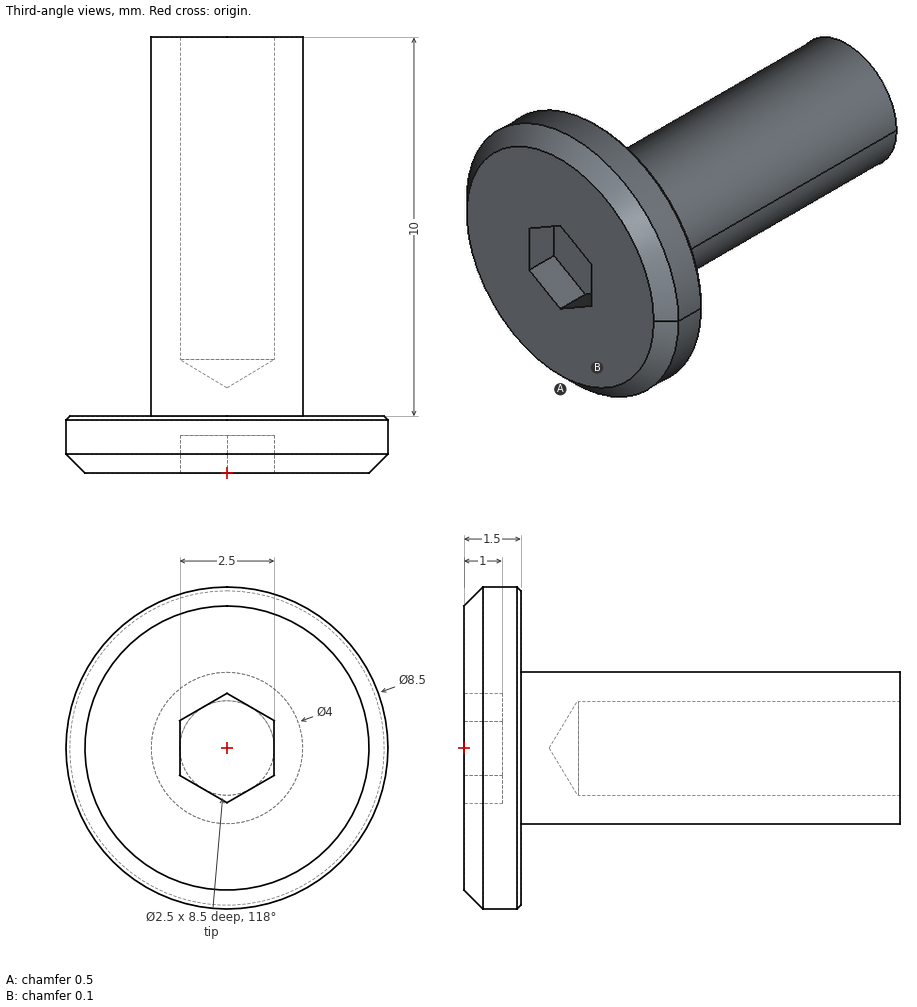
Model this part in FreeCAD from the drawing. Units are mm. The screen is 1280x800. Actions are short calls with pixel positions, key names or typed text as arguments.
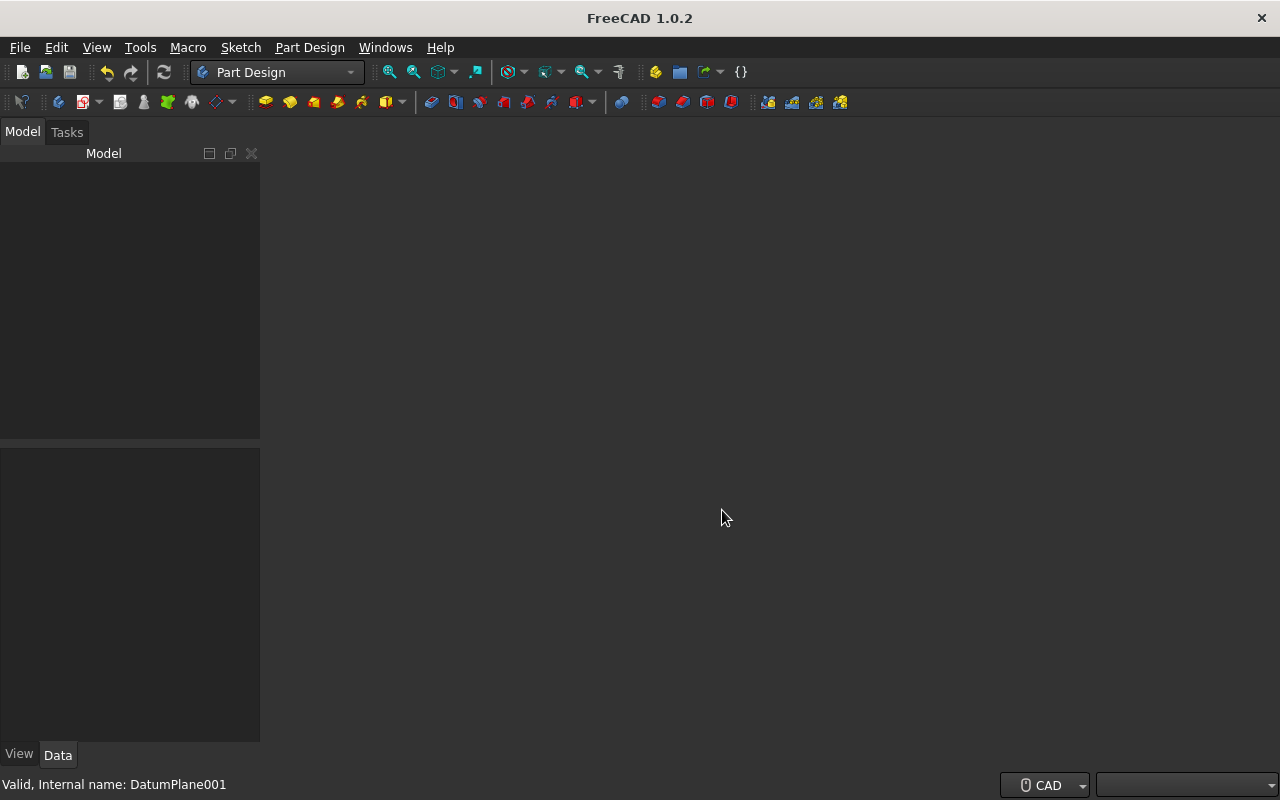
click(22, 72)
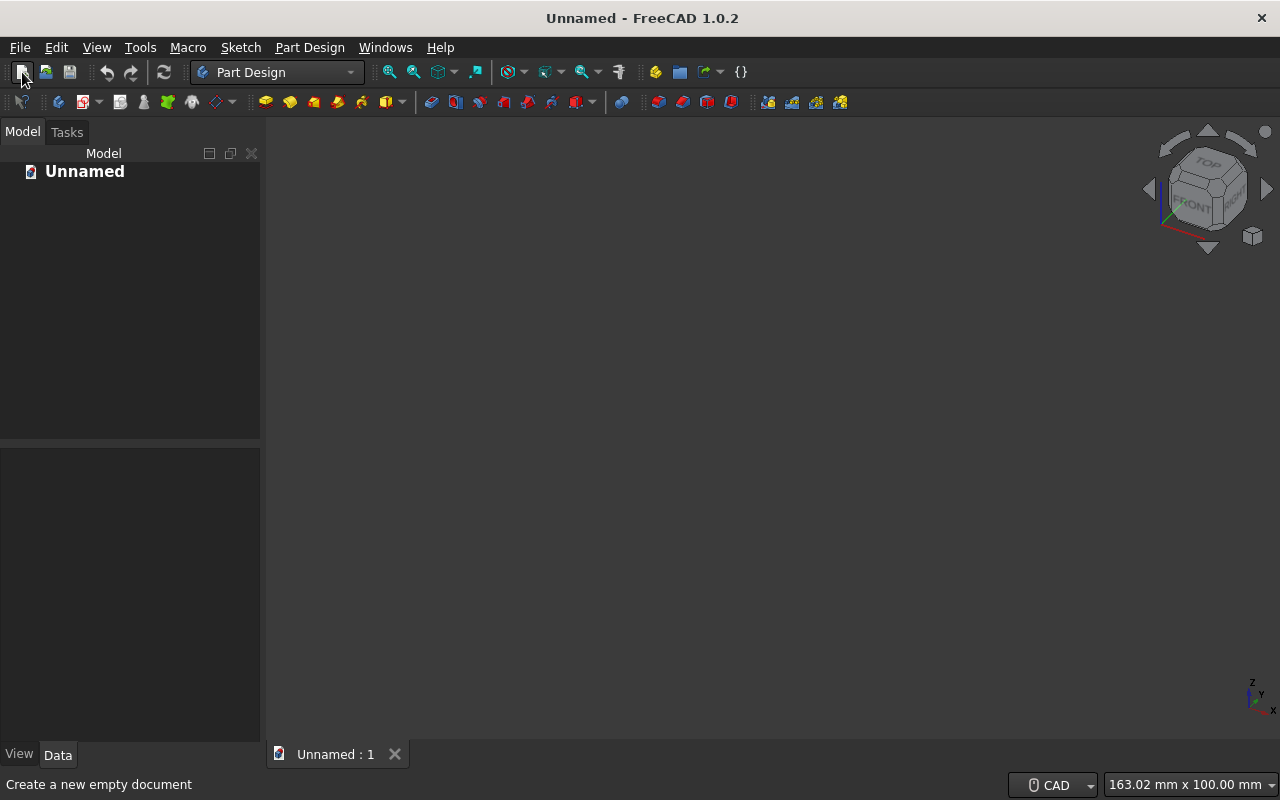
click(84, 102)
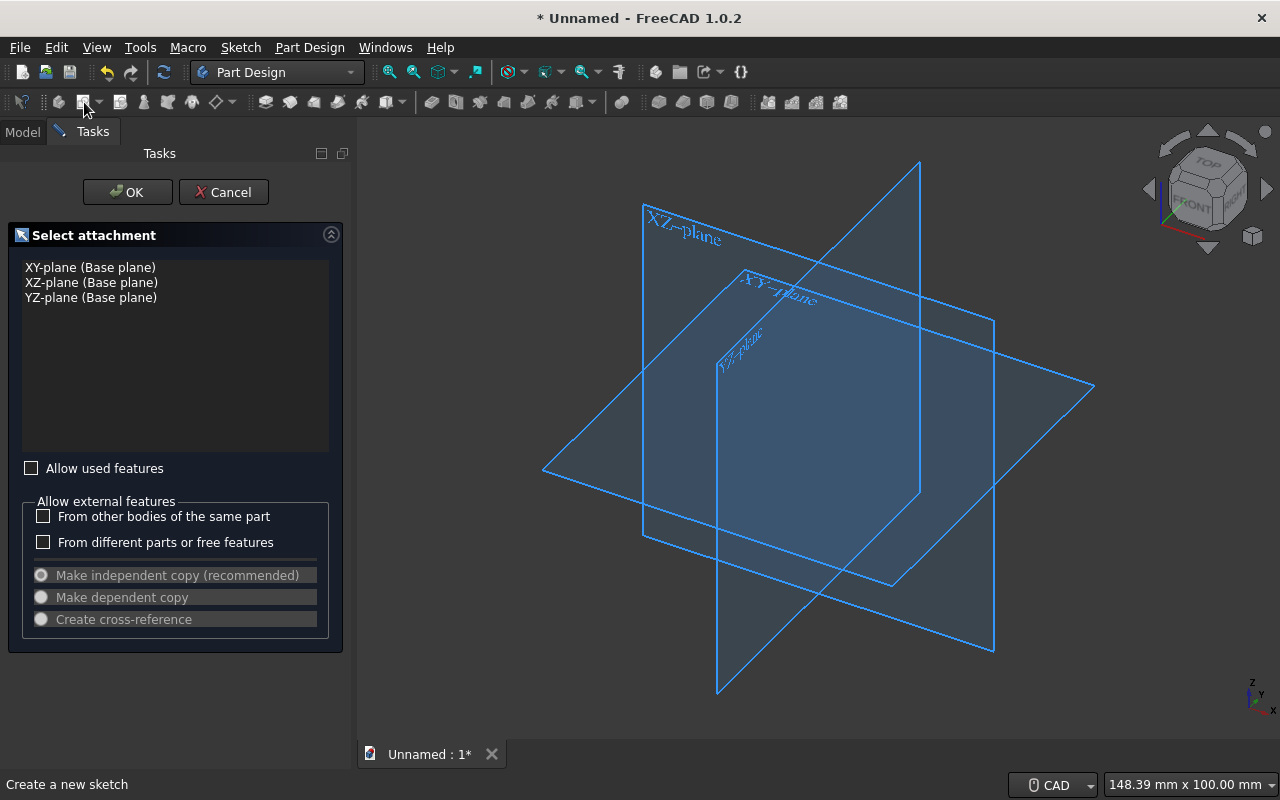
click(82, 282)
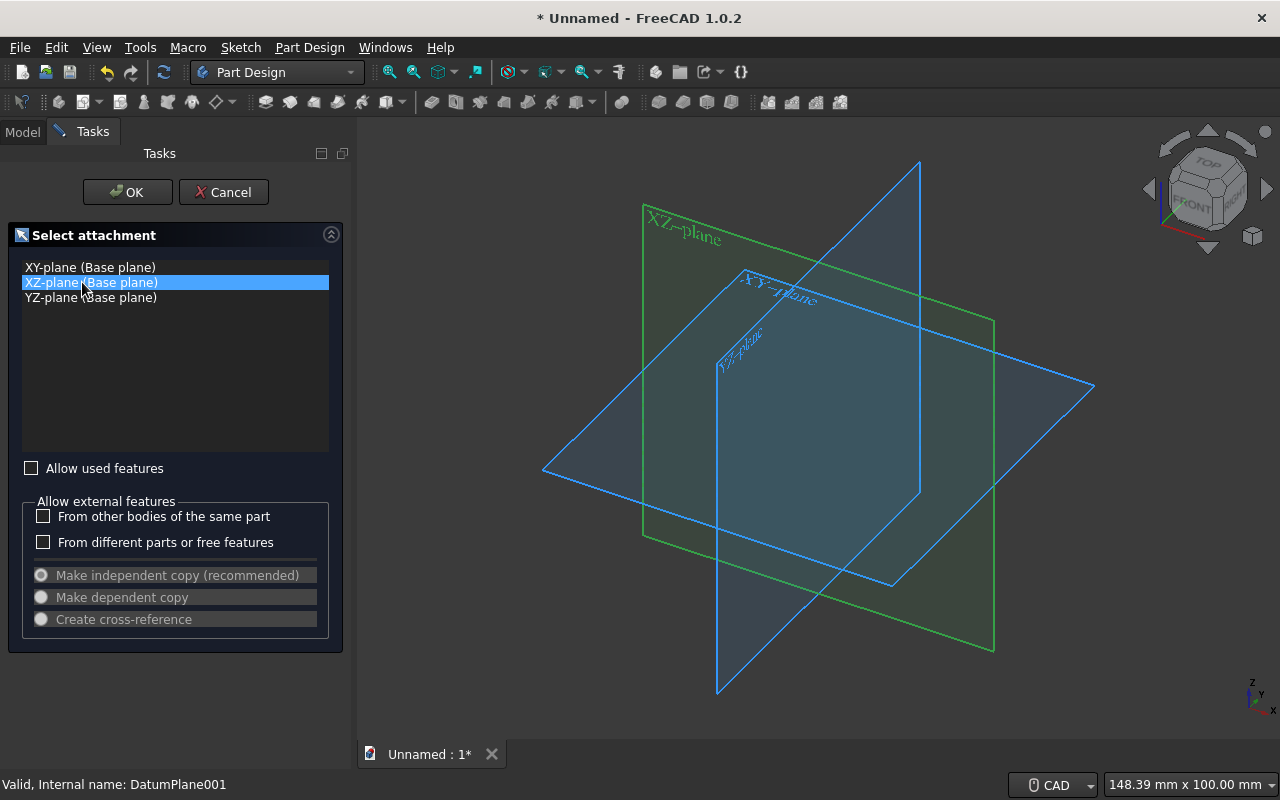
click(128, 192)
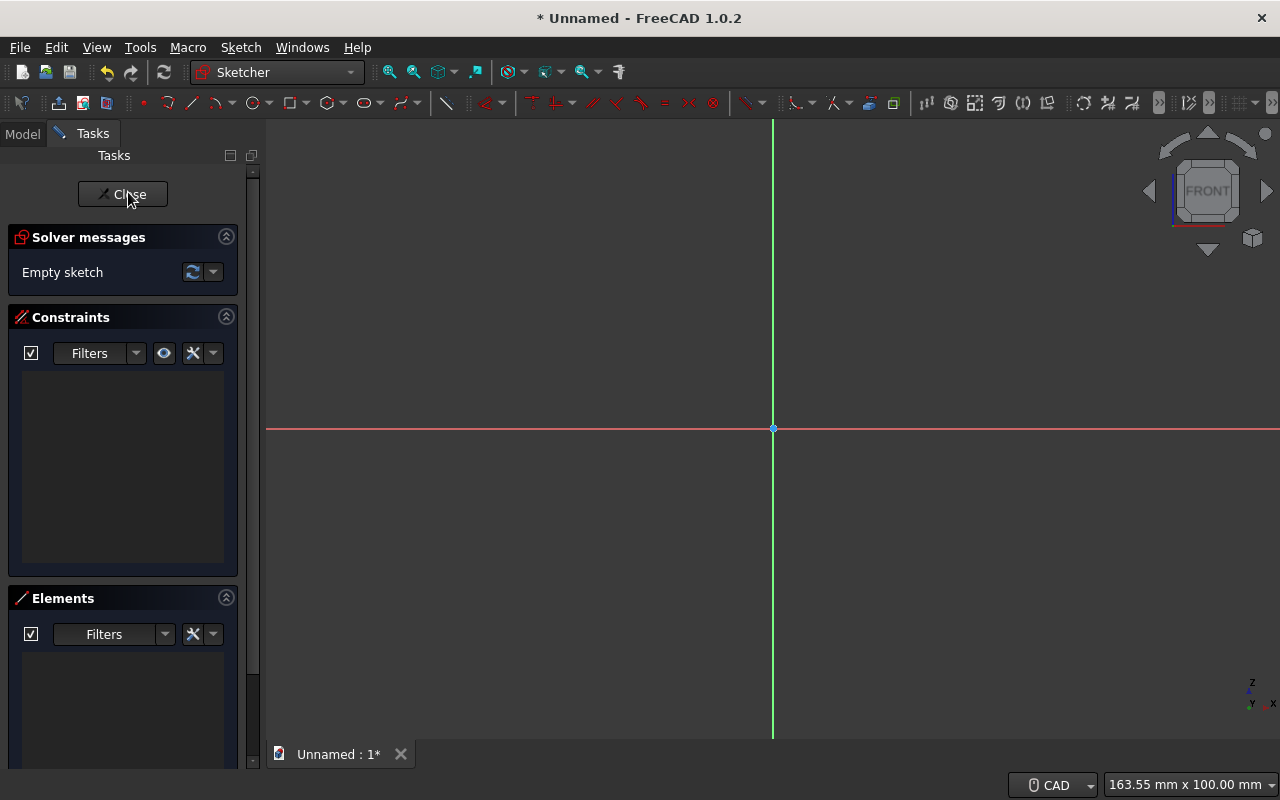
scroll(784, 429, up, 10)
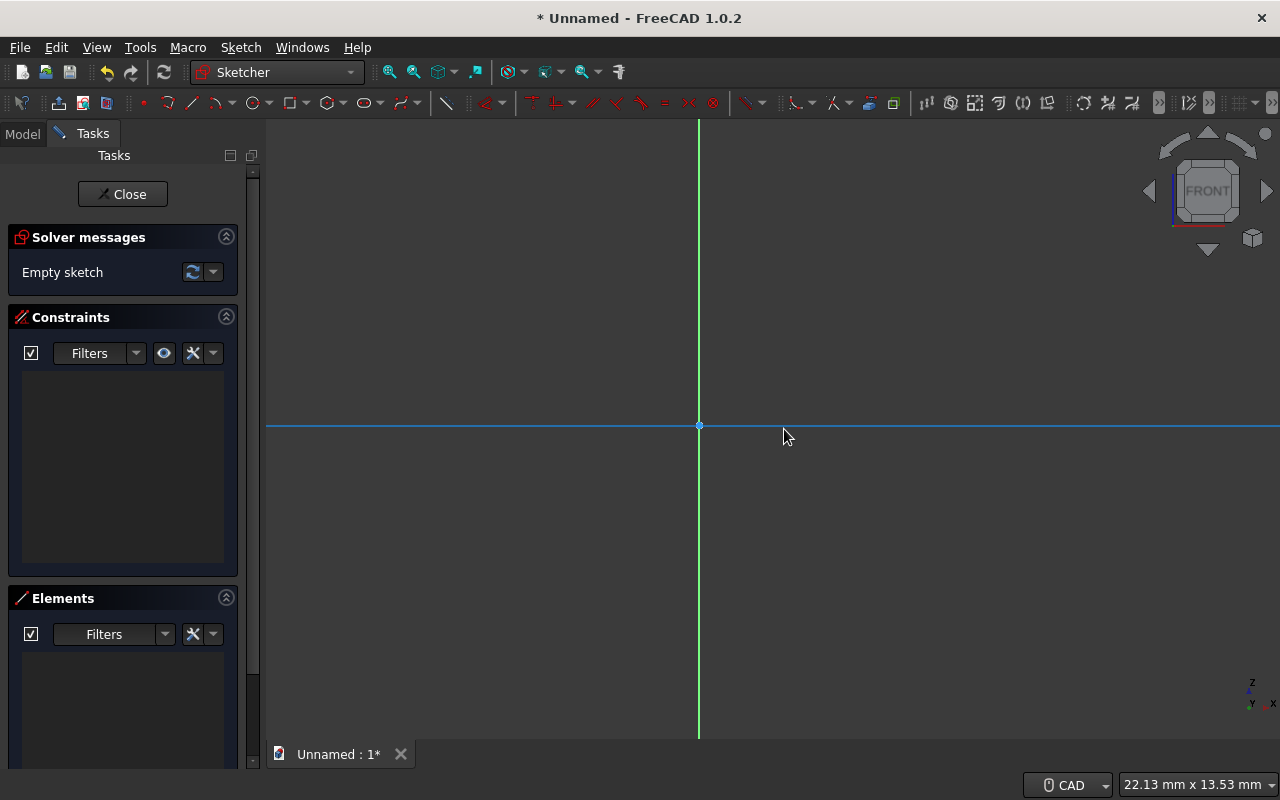
key(g)
key(c)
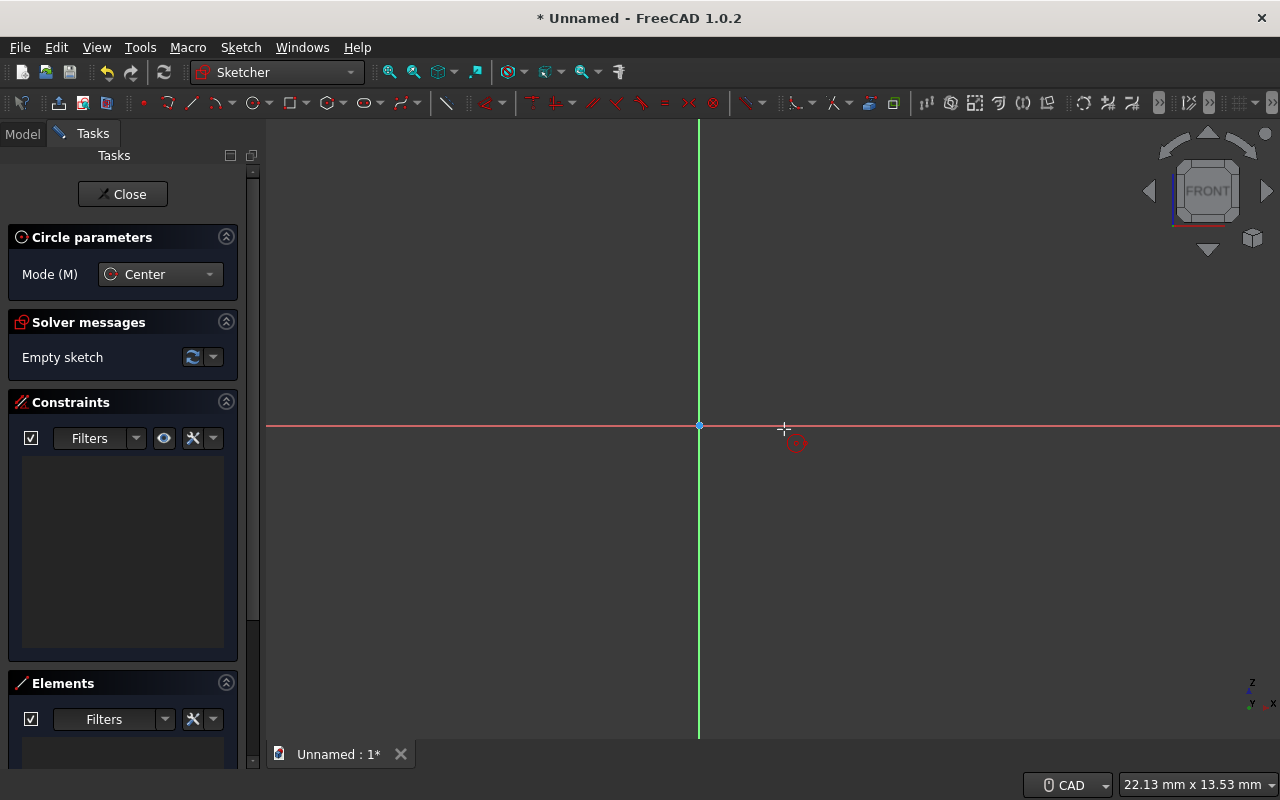
click(699, 426)
move(837, 288)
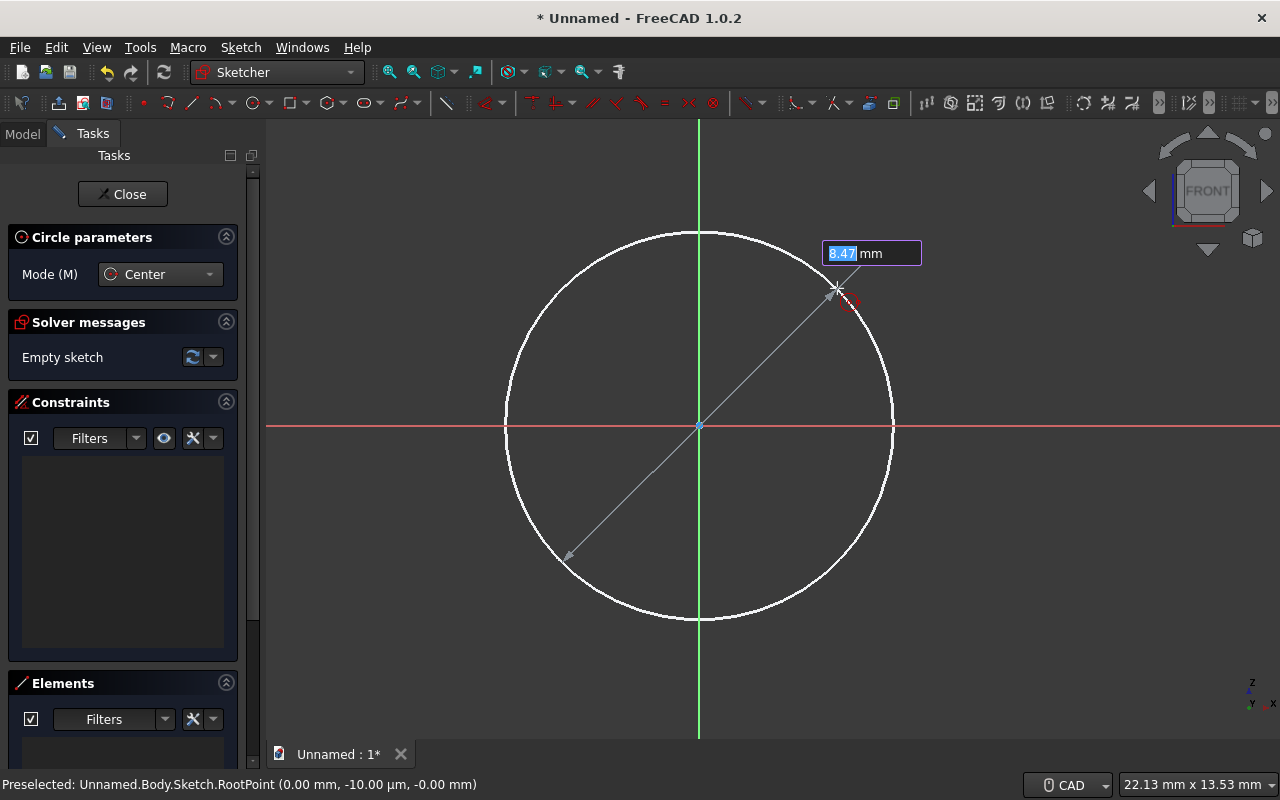
text(8.5)
key(Return)
key(Escape)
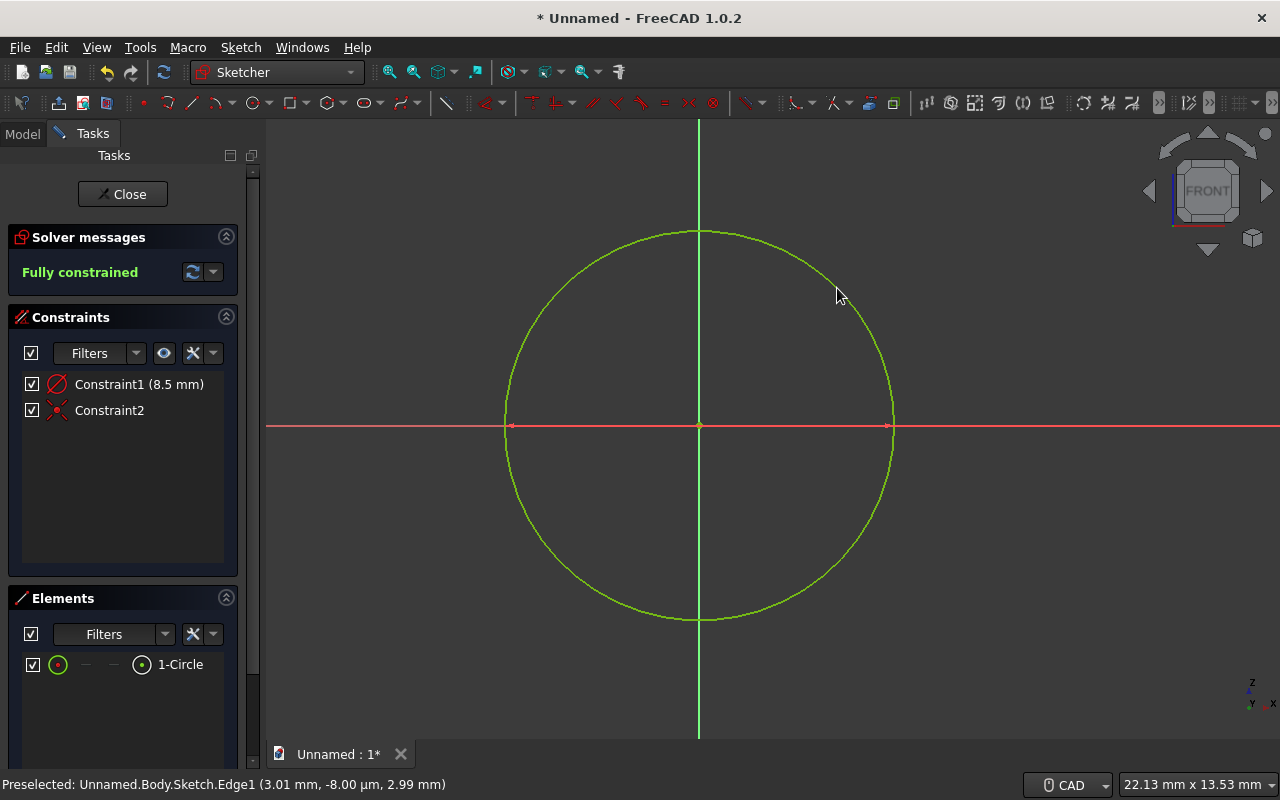
click(123, 194)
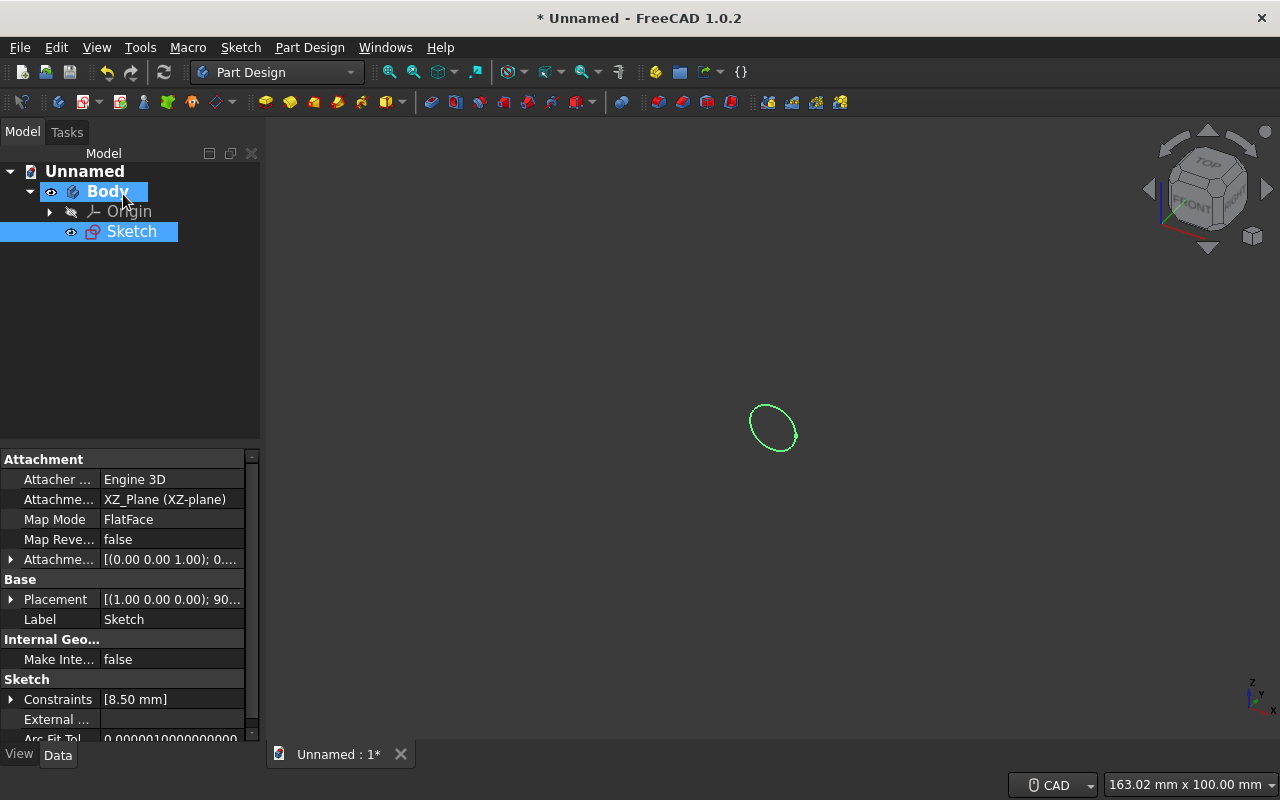
click(266, 102)